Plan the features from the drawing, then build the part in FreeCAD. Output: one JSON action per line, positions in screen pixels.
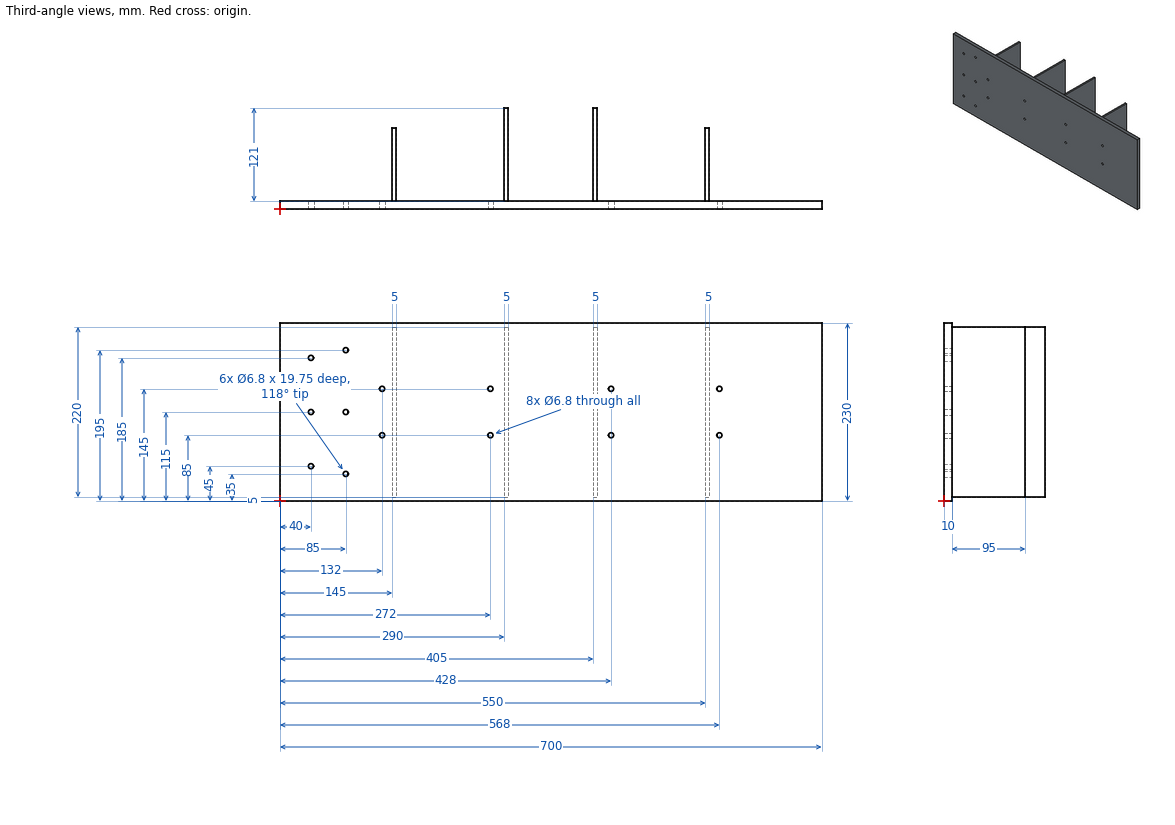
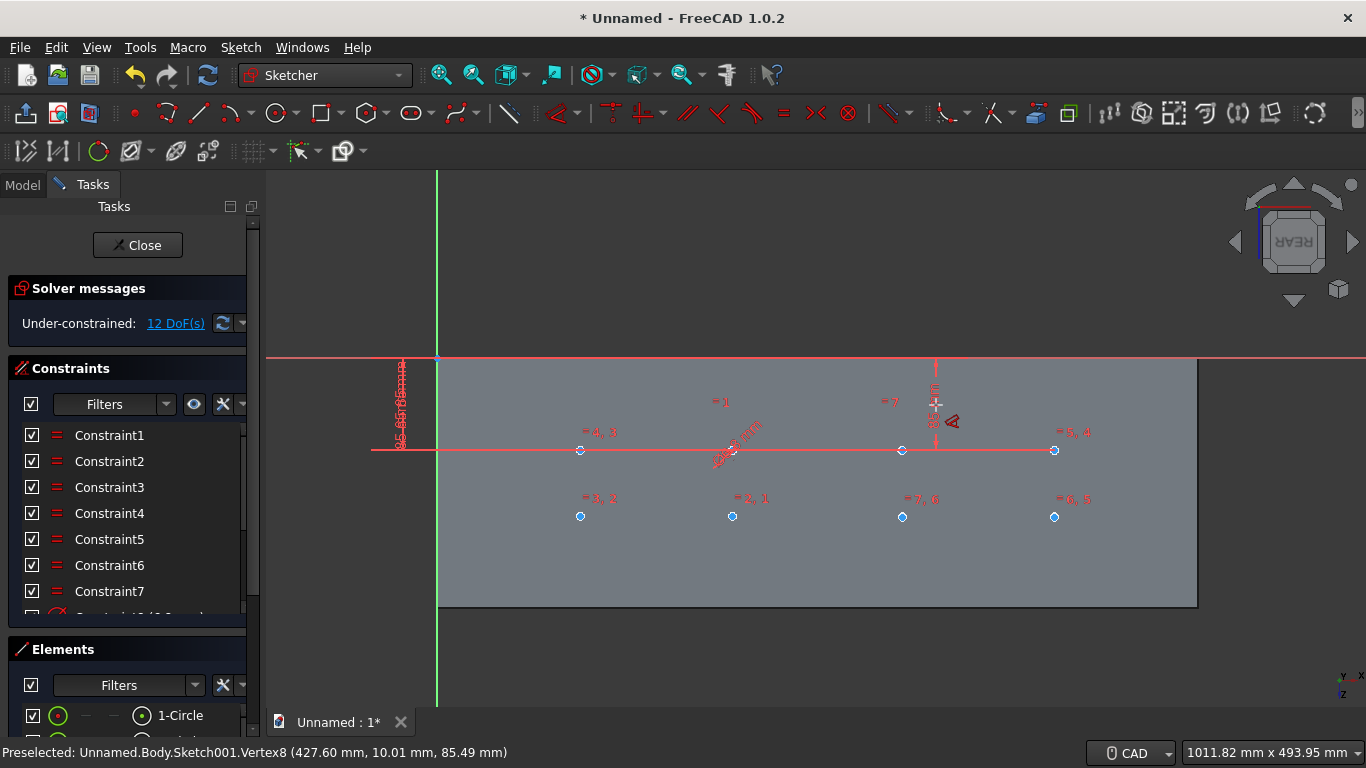
{"action": "left_click", "coordinate": [733, 450]}
{"action": "left_click", "coordinate": [585, 324]}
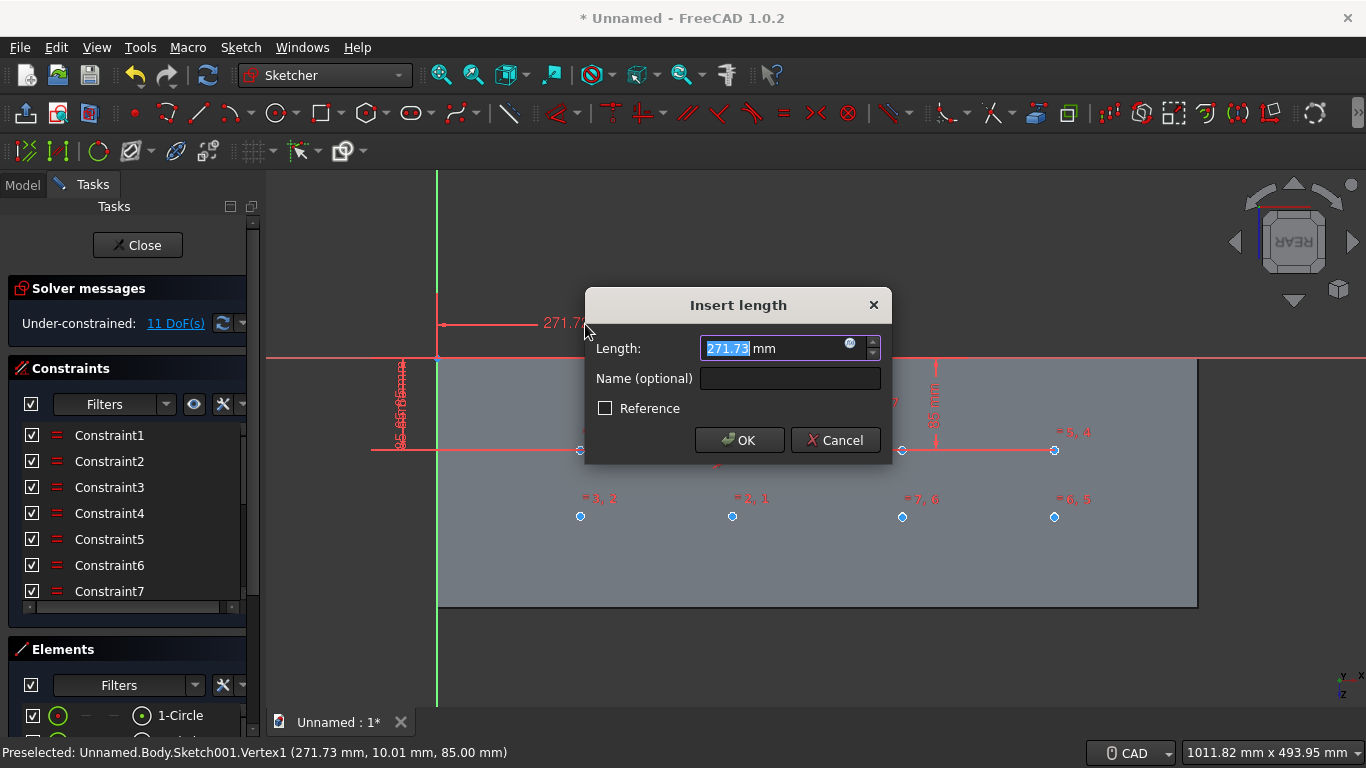
{"action": "type", "text": "272"}
{"action": "key", "text": "Return"}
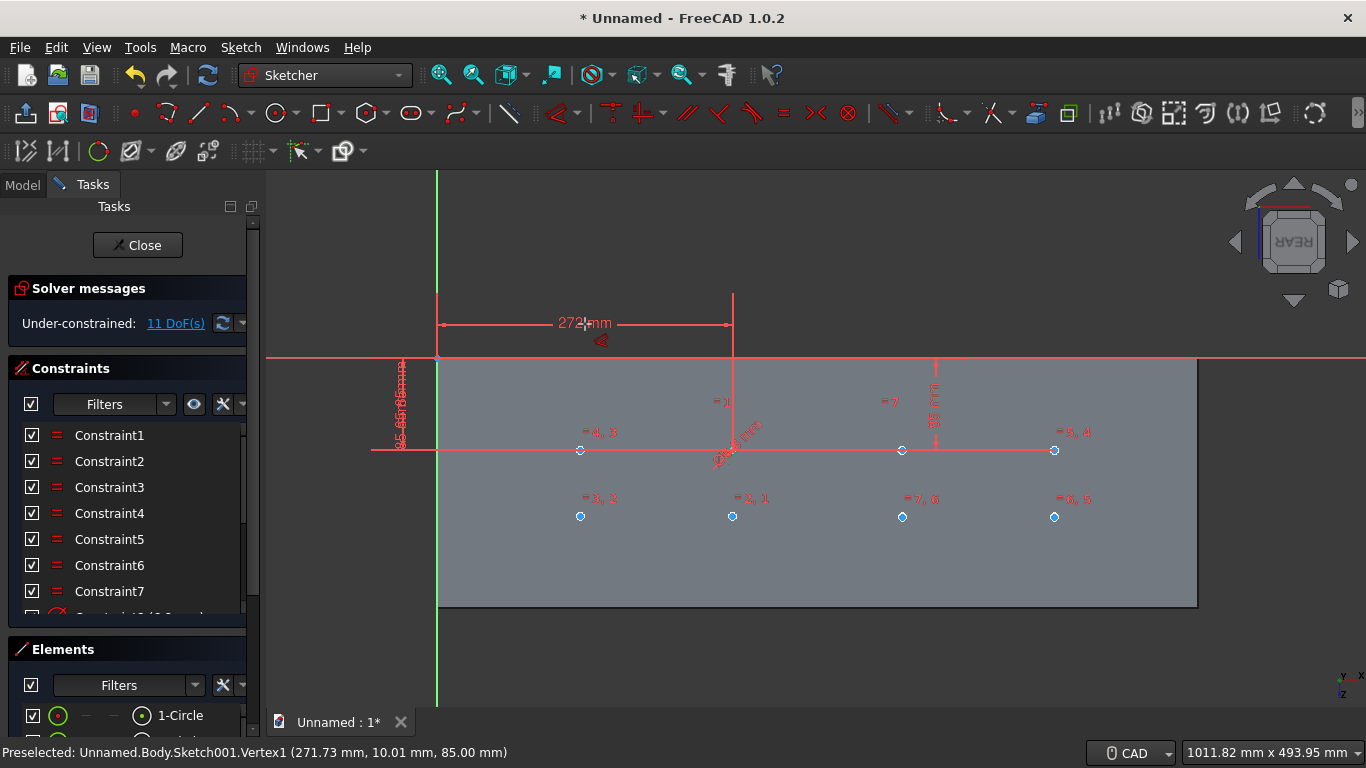
{"action": "left_click", "coordinate": [733, 516]}
{"action": "left_click", "coordinate": [481, 324]}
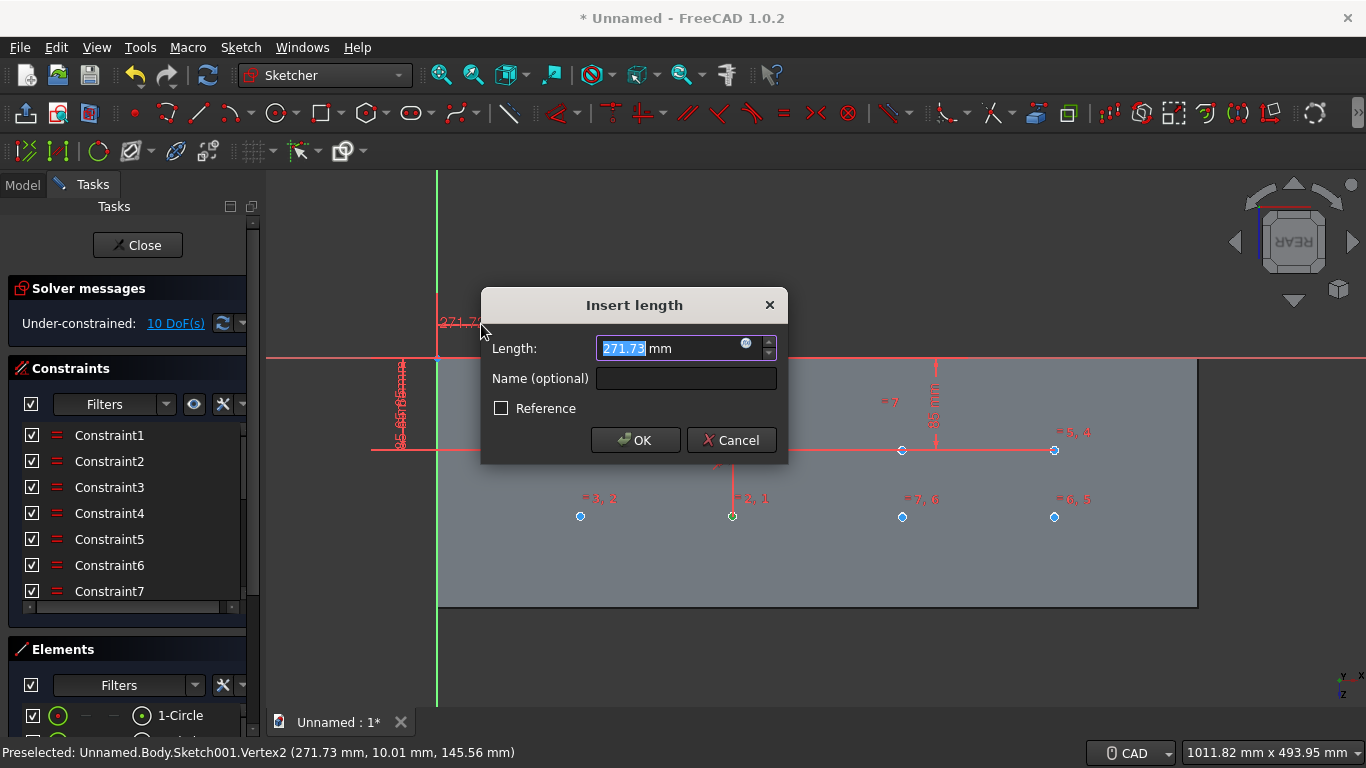
{"action": "type", "text": "272"}
{"action": "key", "text": "Return"}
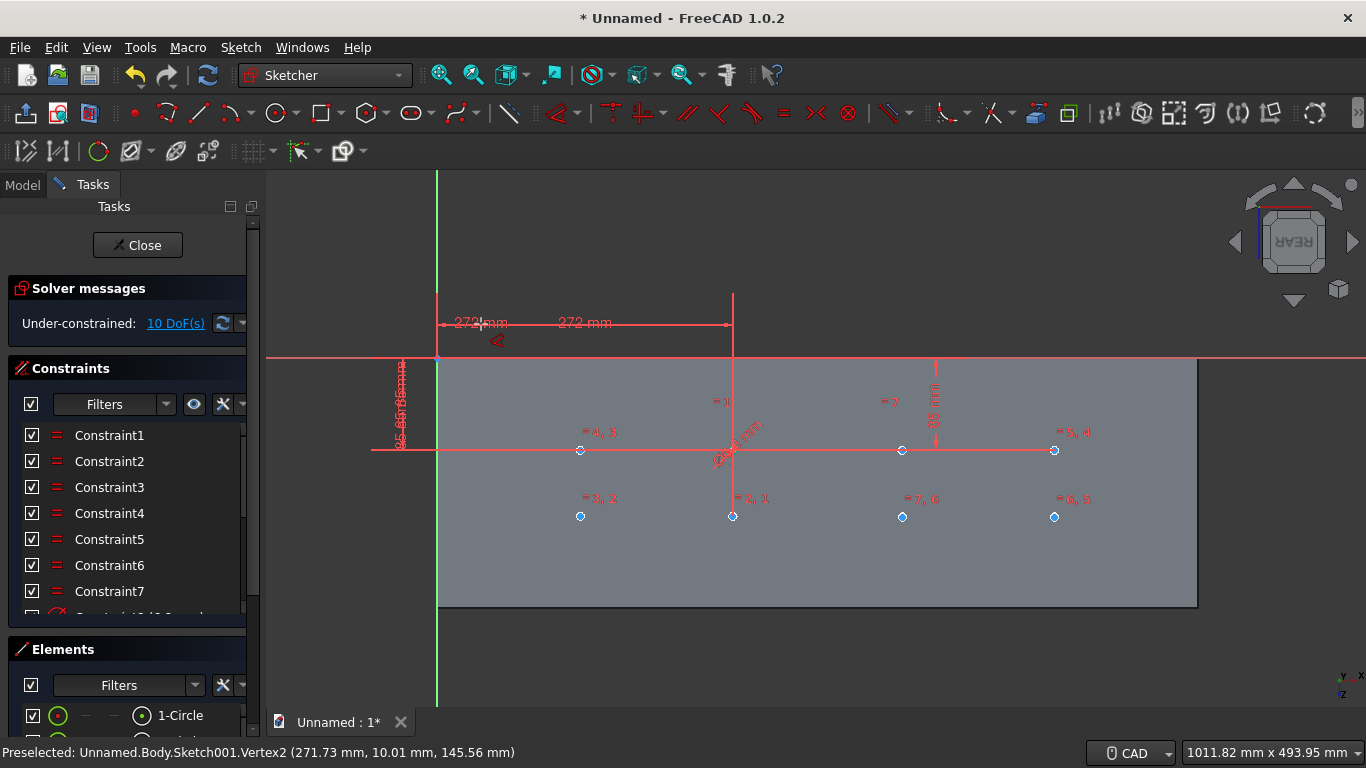
{"action": "left_click", "coordinate": [733, 516]}
{"action": "left_click", "coordinate": [403, 474]}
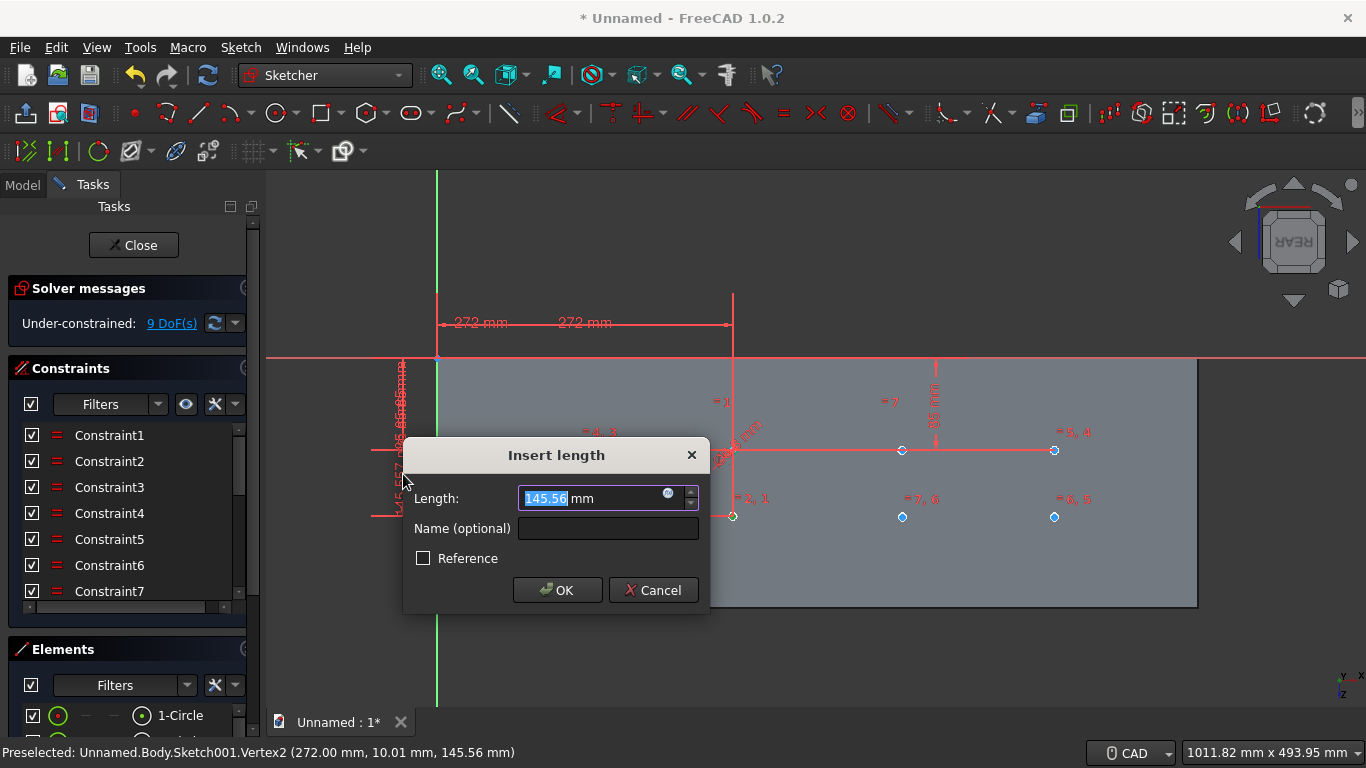
{"action": "type", "text": "145"}
{"action": "key", "text": "Return"}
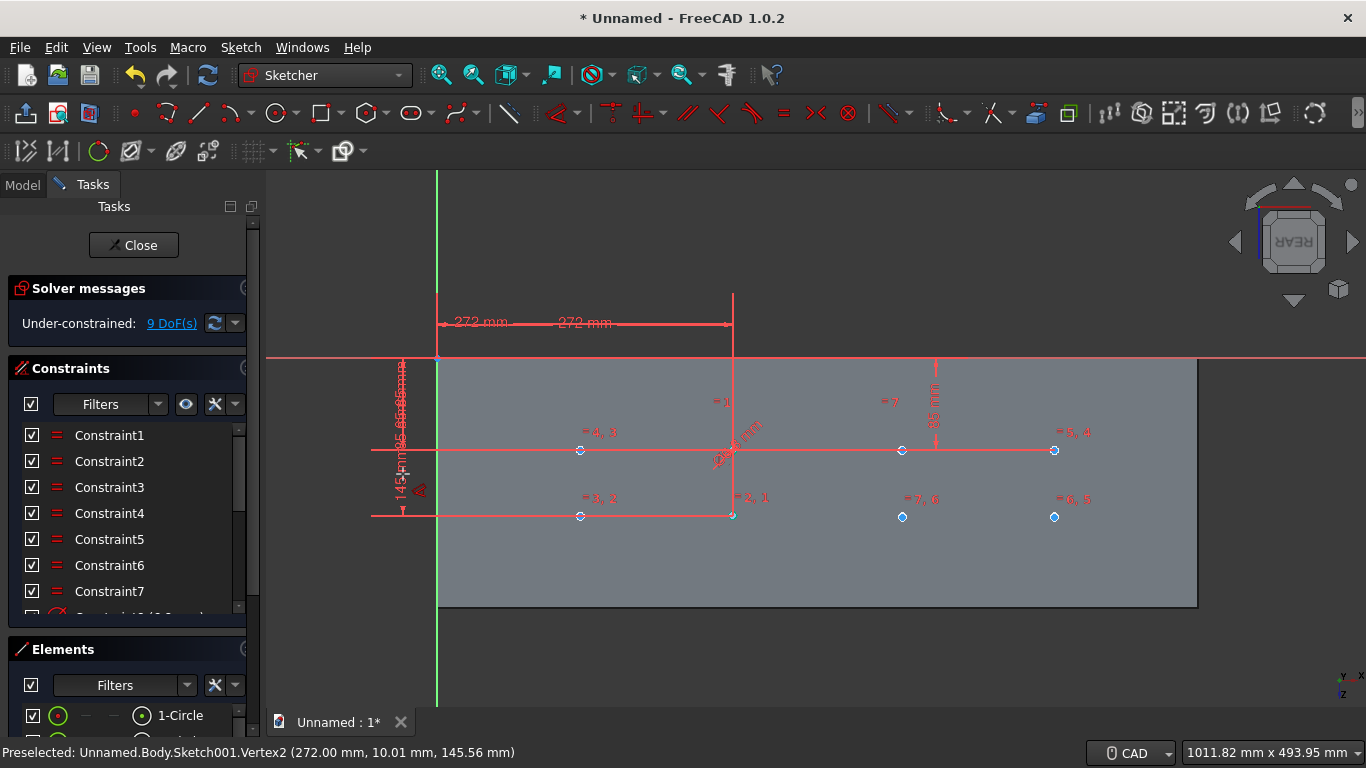
{"action": "left_click", "coordinate": [580, 516]}
{"action": "left_click", "coordinate": [509, 550]}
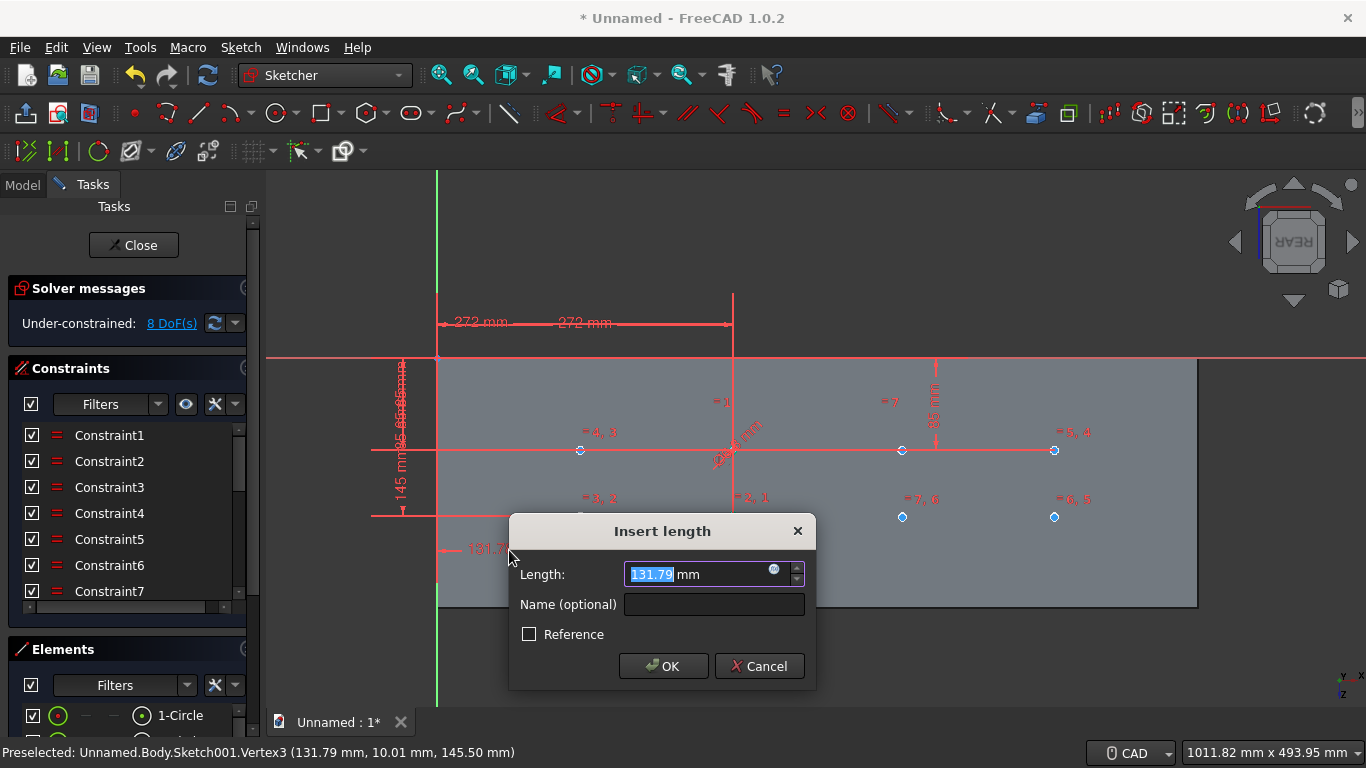
{"action": "type", "text": "132"}
{"action": "key", "text": "Return"}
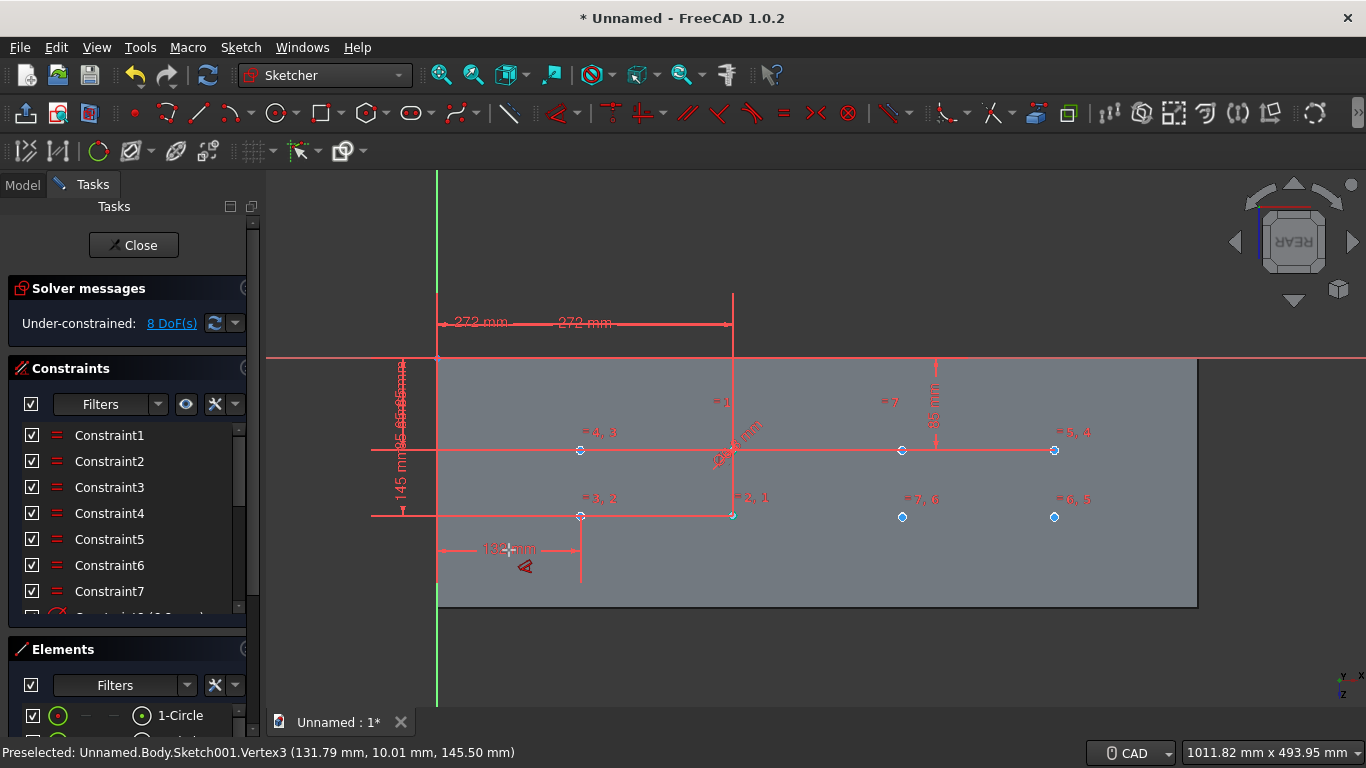
{"action": "left_click", "coordinate": [581, 516]}
{"action": "left_click", "coordinate": [615, 437]}